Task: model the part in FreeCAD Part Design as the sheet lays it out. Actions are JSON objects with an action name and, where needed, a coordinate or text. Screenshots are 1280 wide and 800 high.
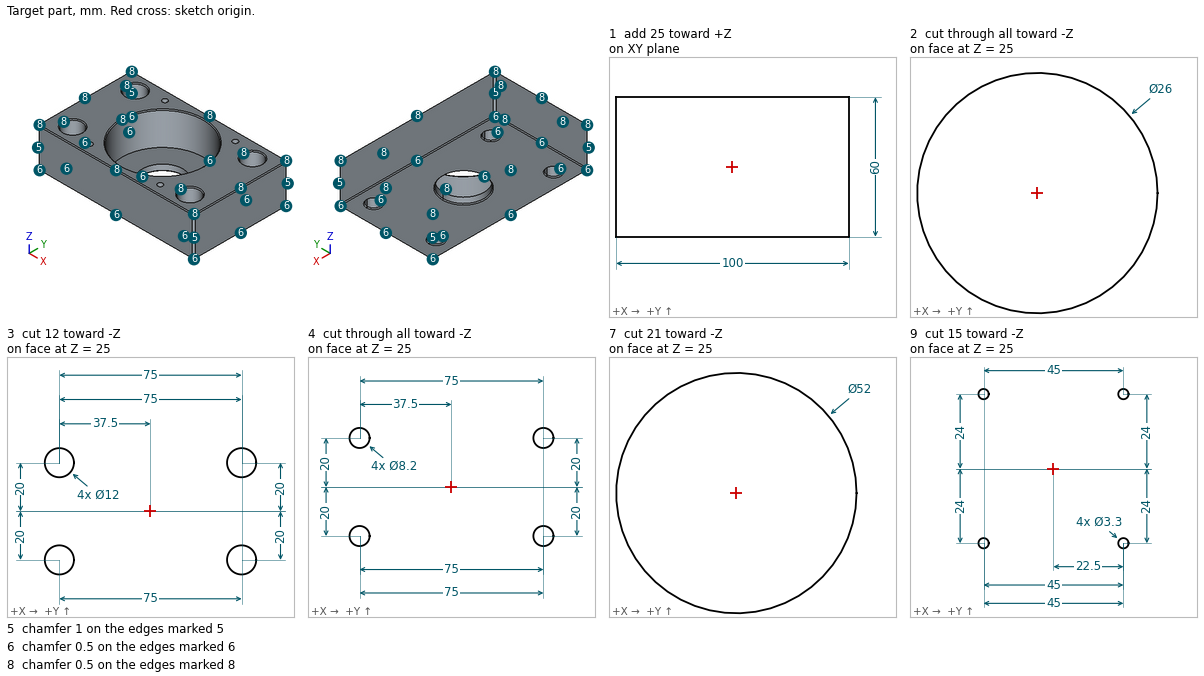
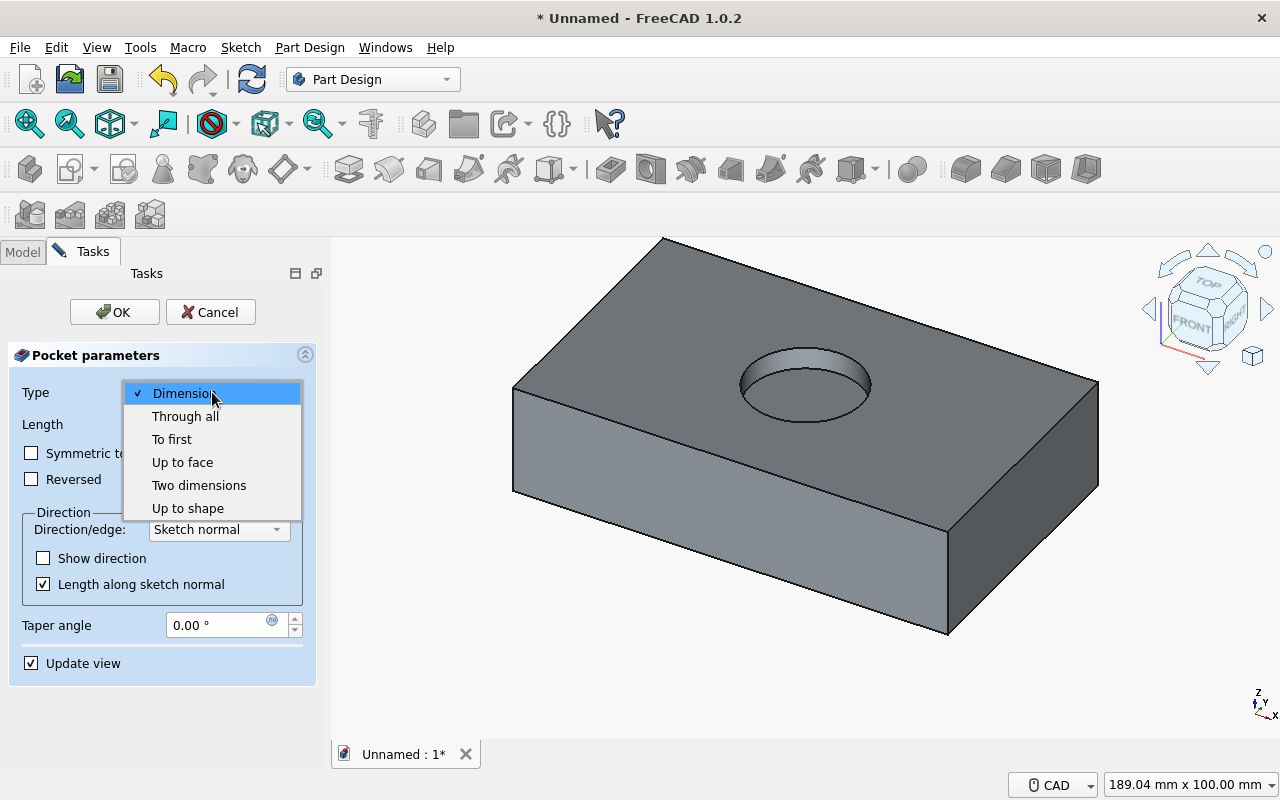
{"action": "left_click", "coordinate": [212, 416]}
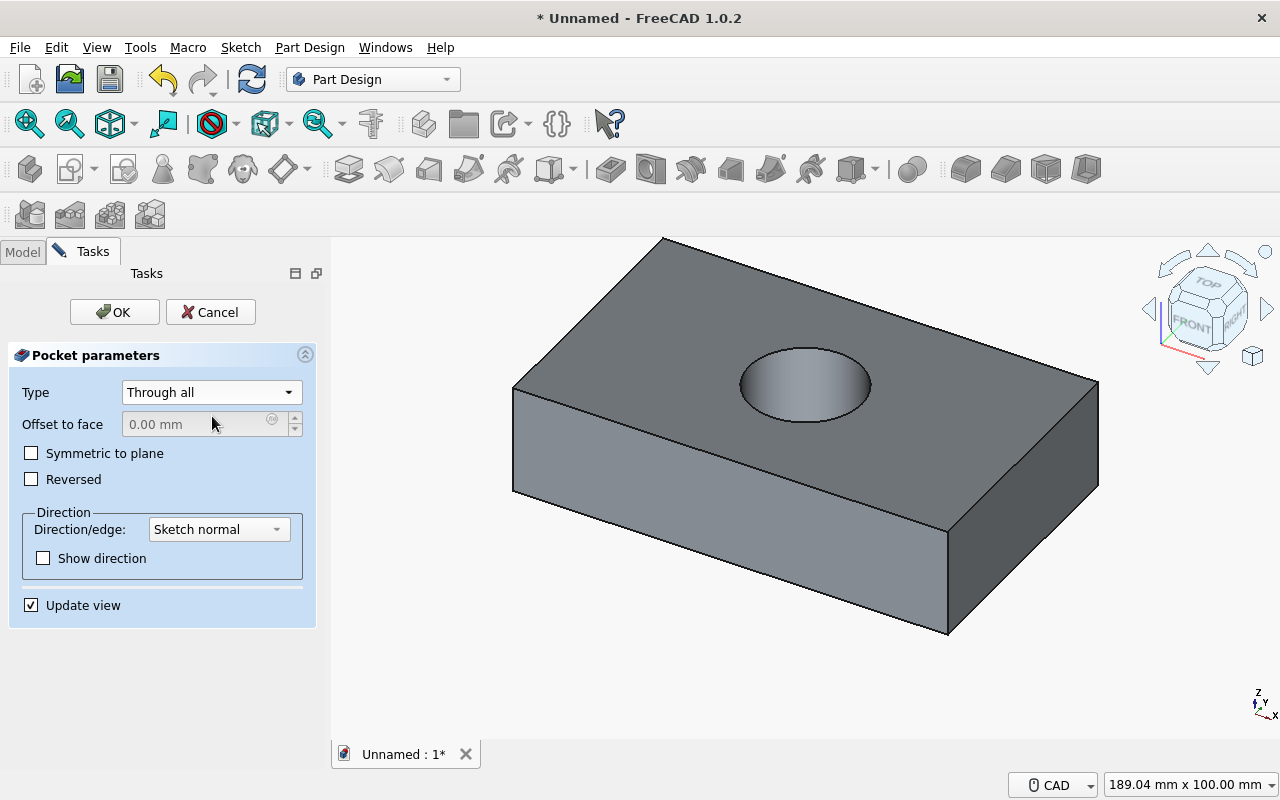
{"action": "left_click", "coordinate": [115, 312]}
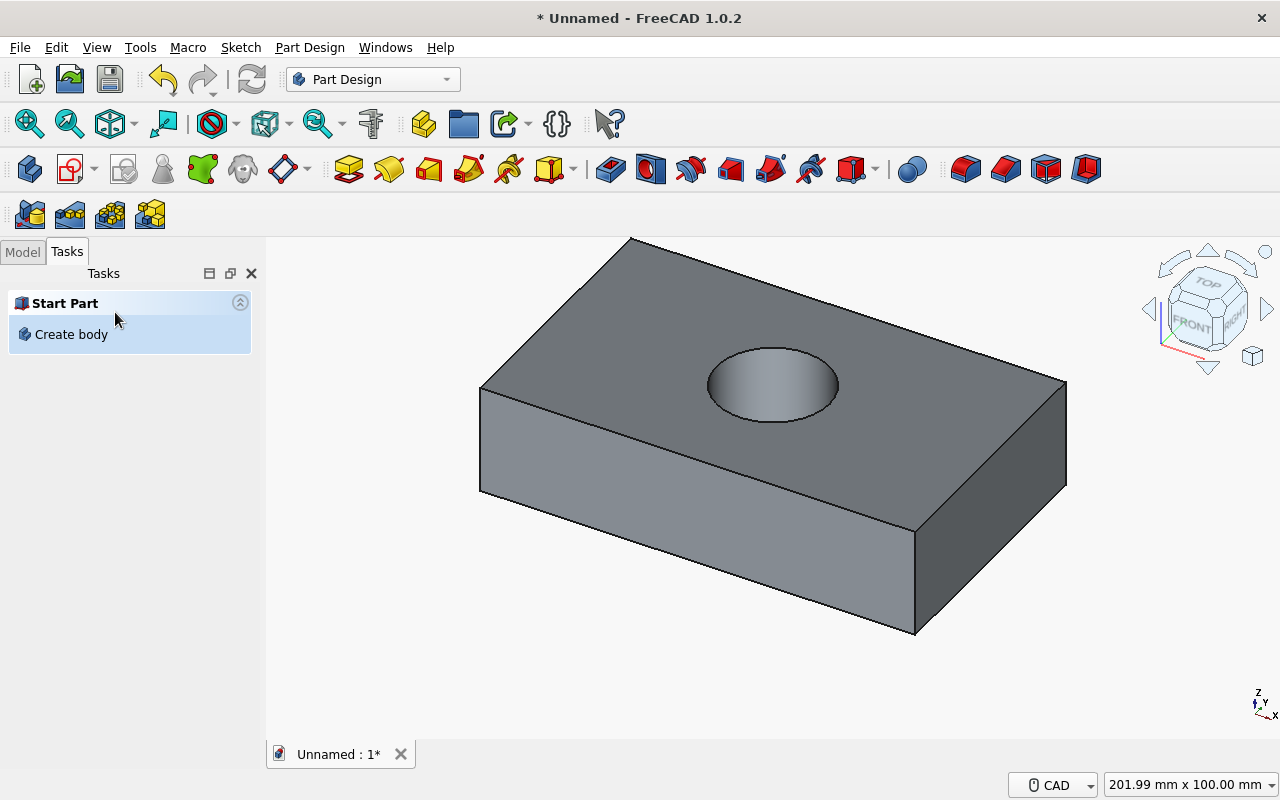
{"action": "left_click", "coordinate": [670, 322]}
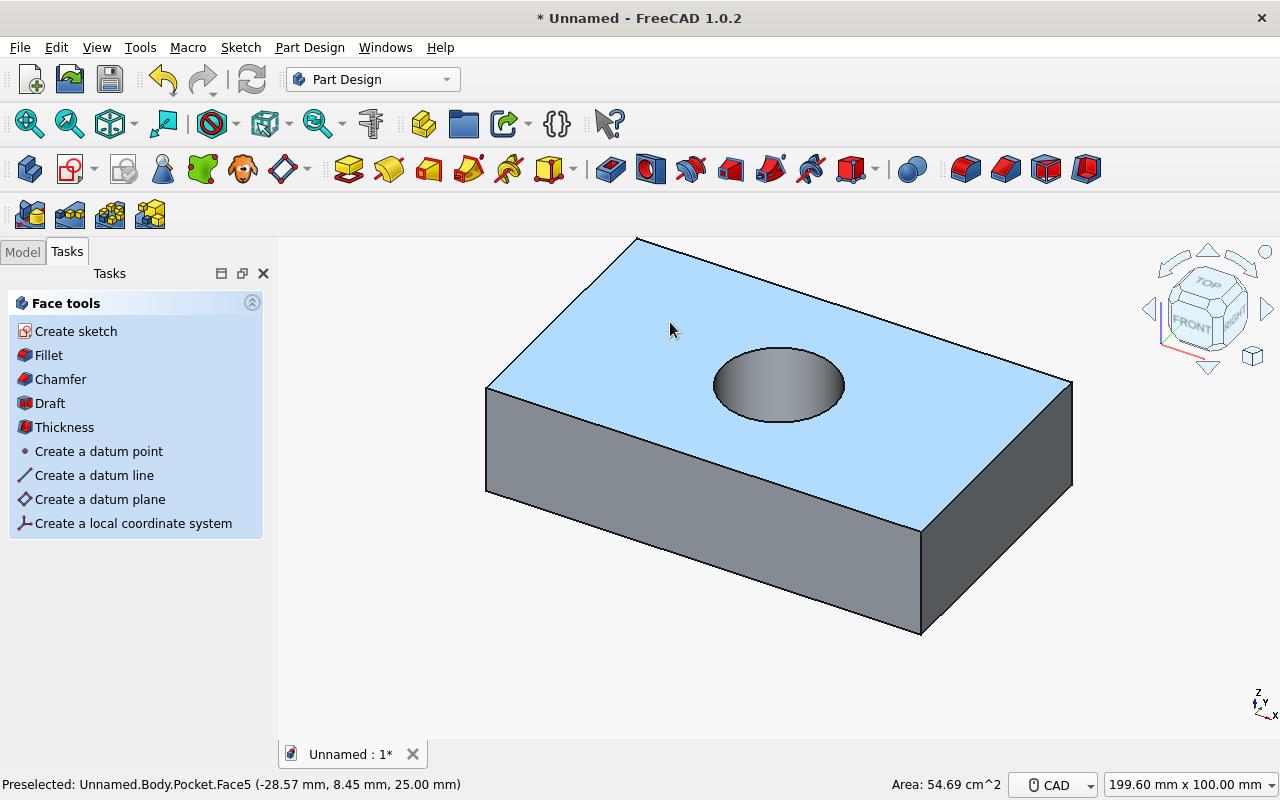
{"action": "left_click", "coordinate": [70, 170]}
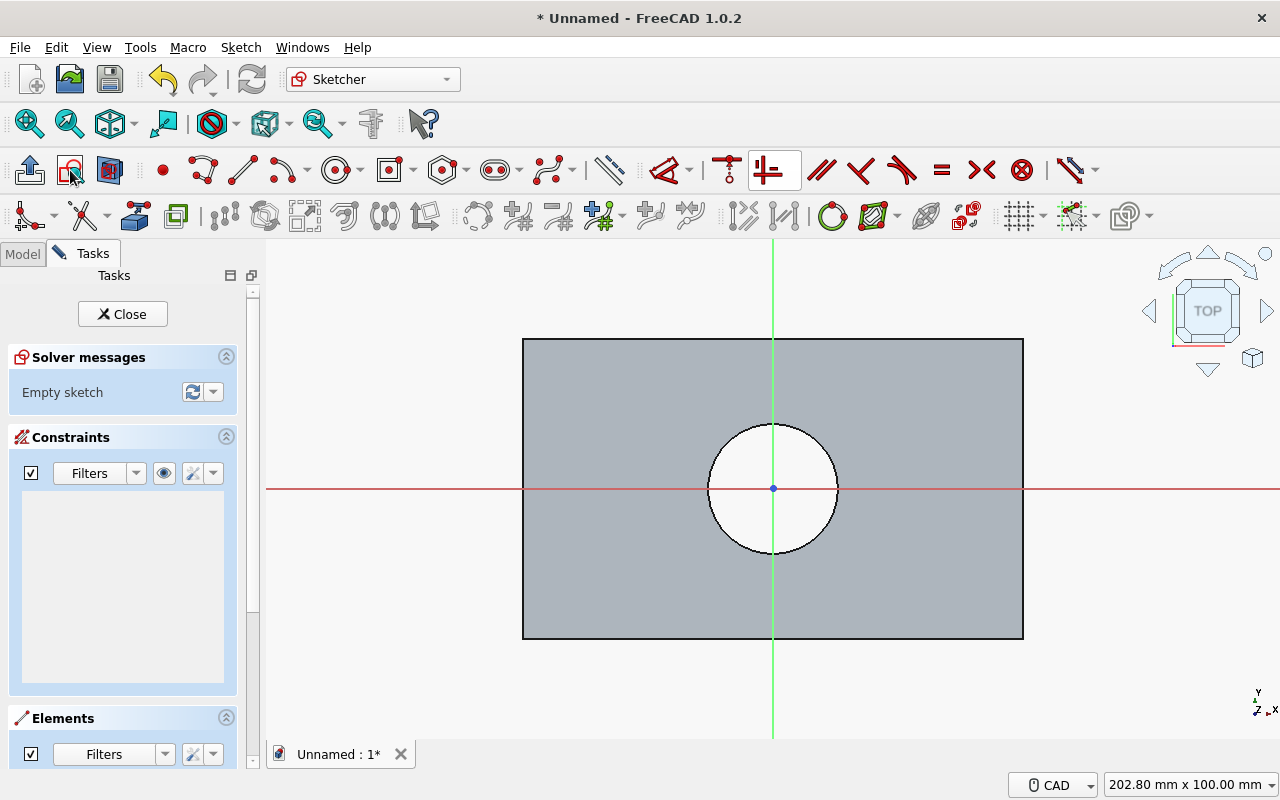
{"action": "key", "text": "g c"}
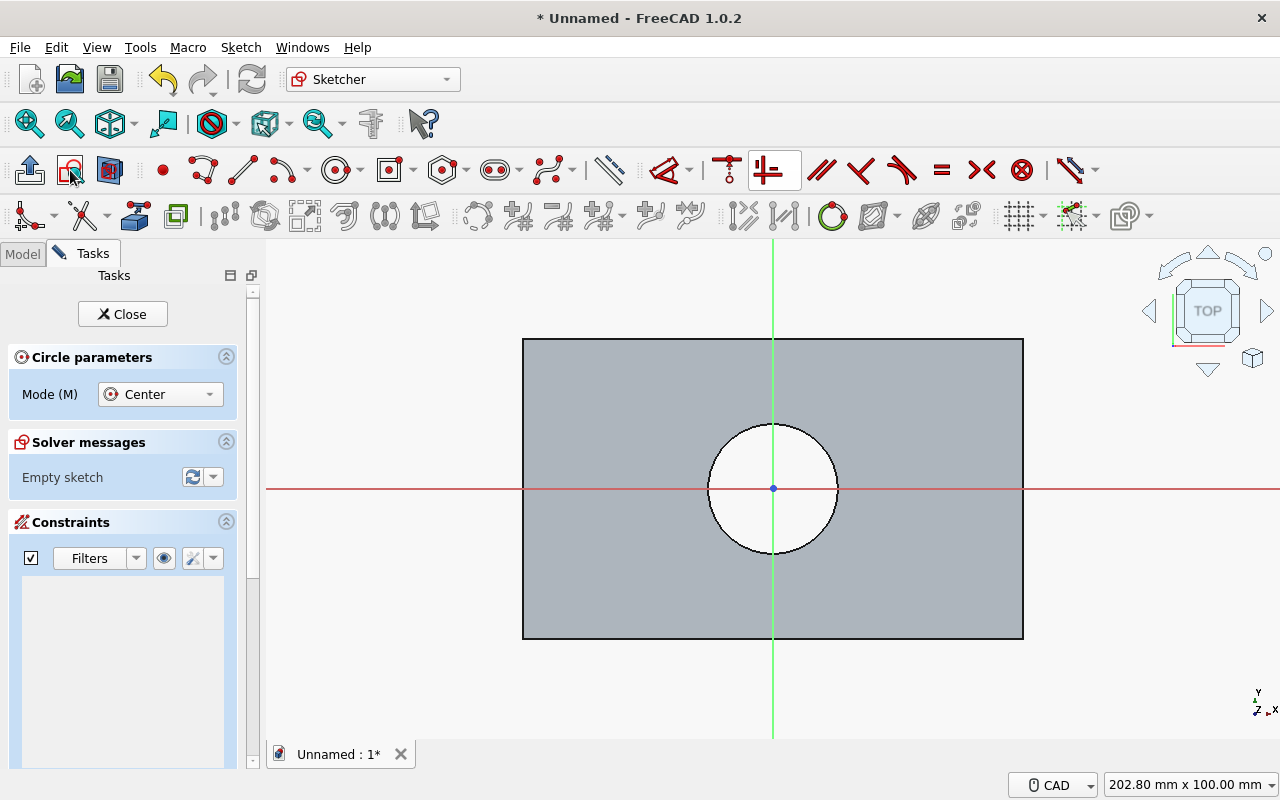
{"action": "left_click", "coordinate": [585, 389]}
{"action": "mouse_move", "coordinate": [607, 368]}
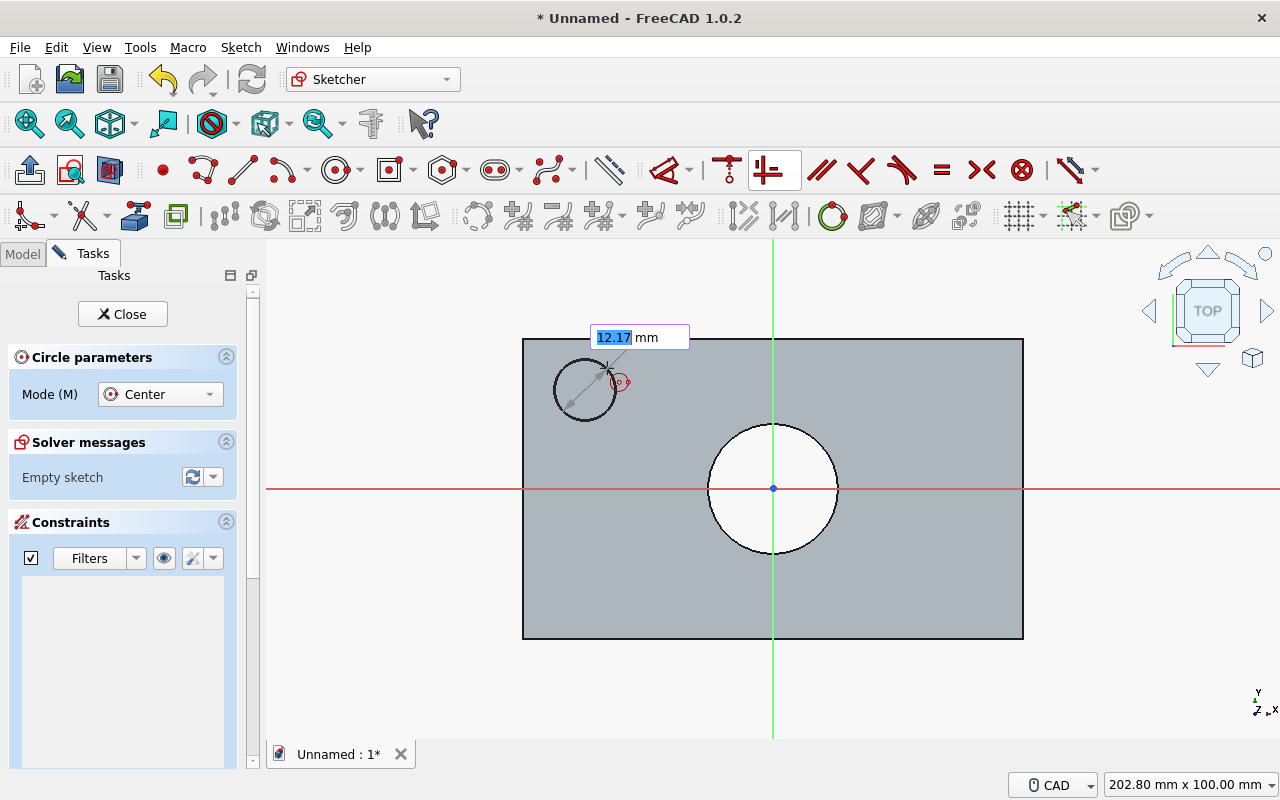
{"action": "type", "text": "12"}
{"action": "key", "text": "Return"}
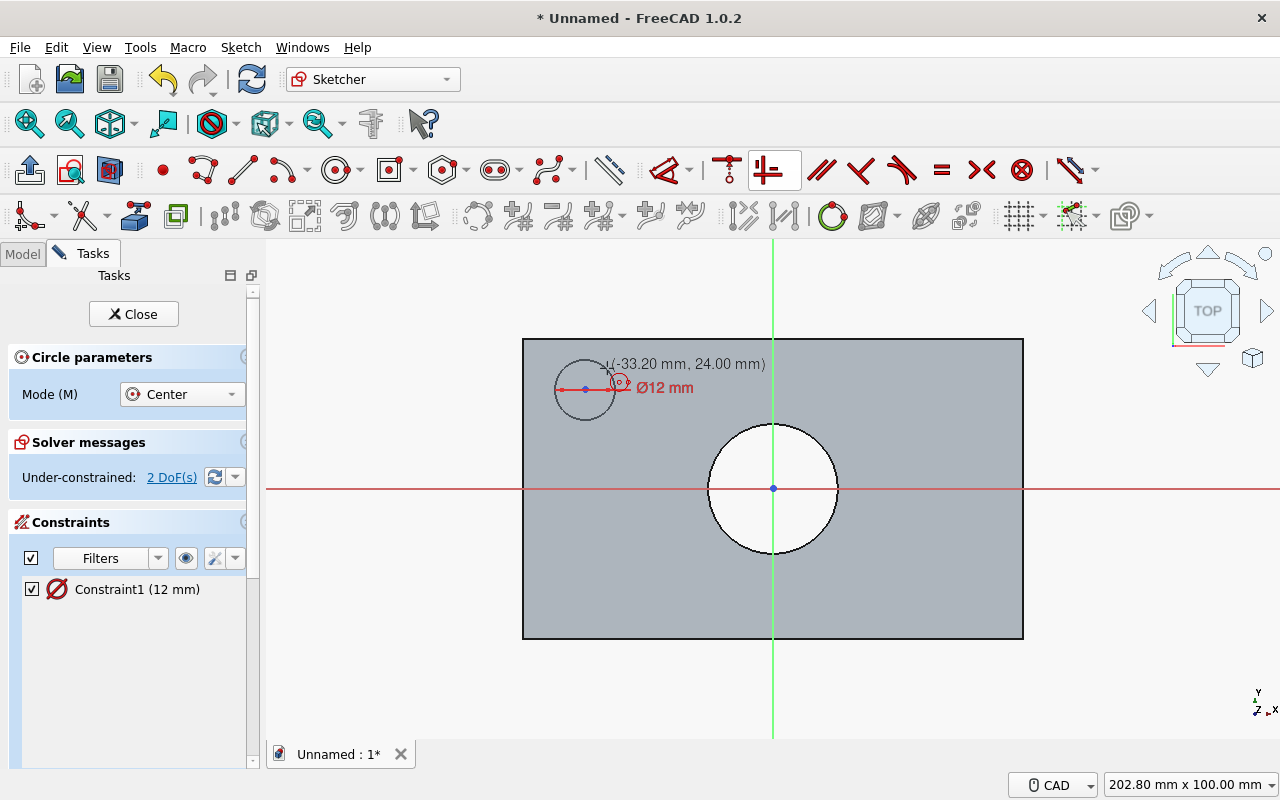
{"action": "left_click", "coordinate": [585, 589]}
{"action": "mouse_move", "coordinate": [607, 568]}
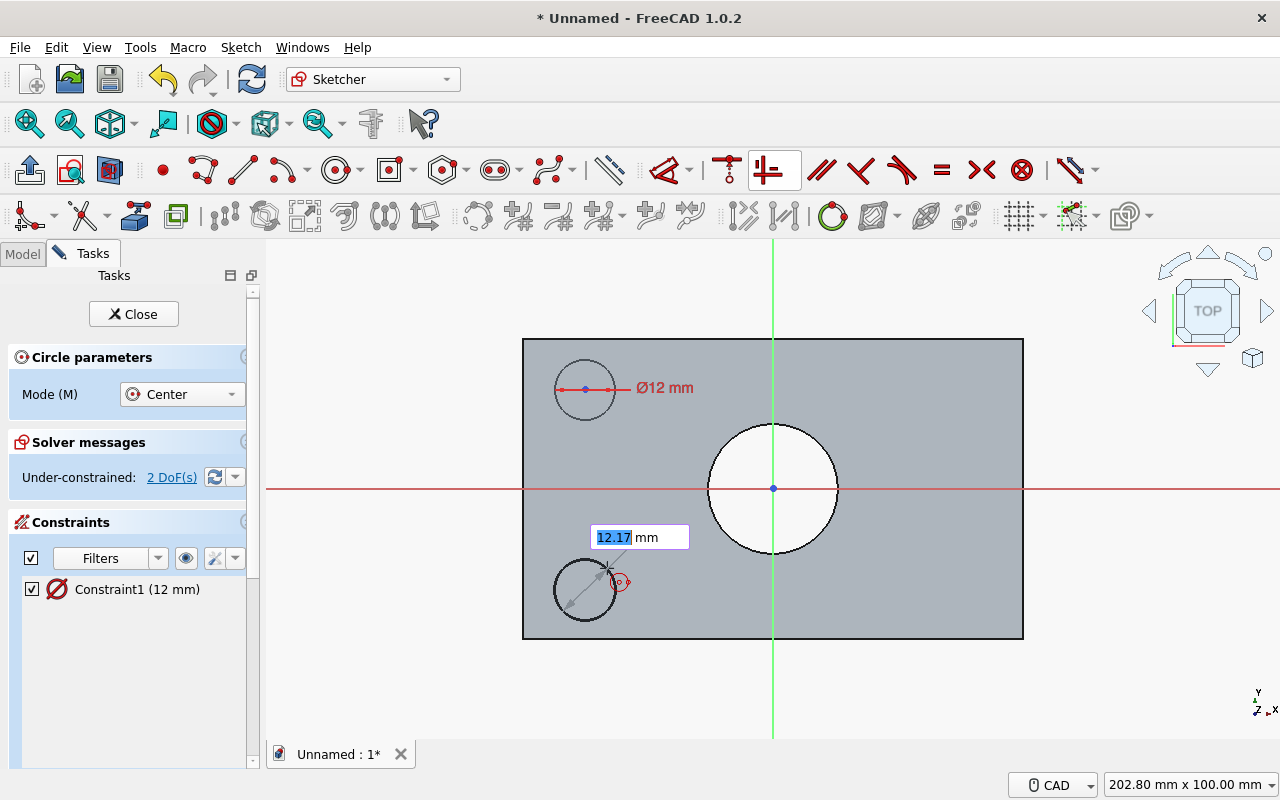
{"action": "type", "text": "12"}
{"action": "key", "text": "Return"}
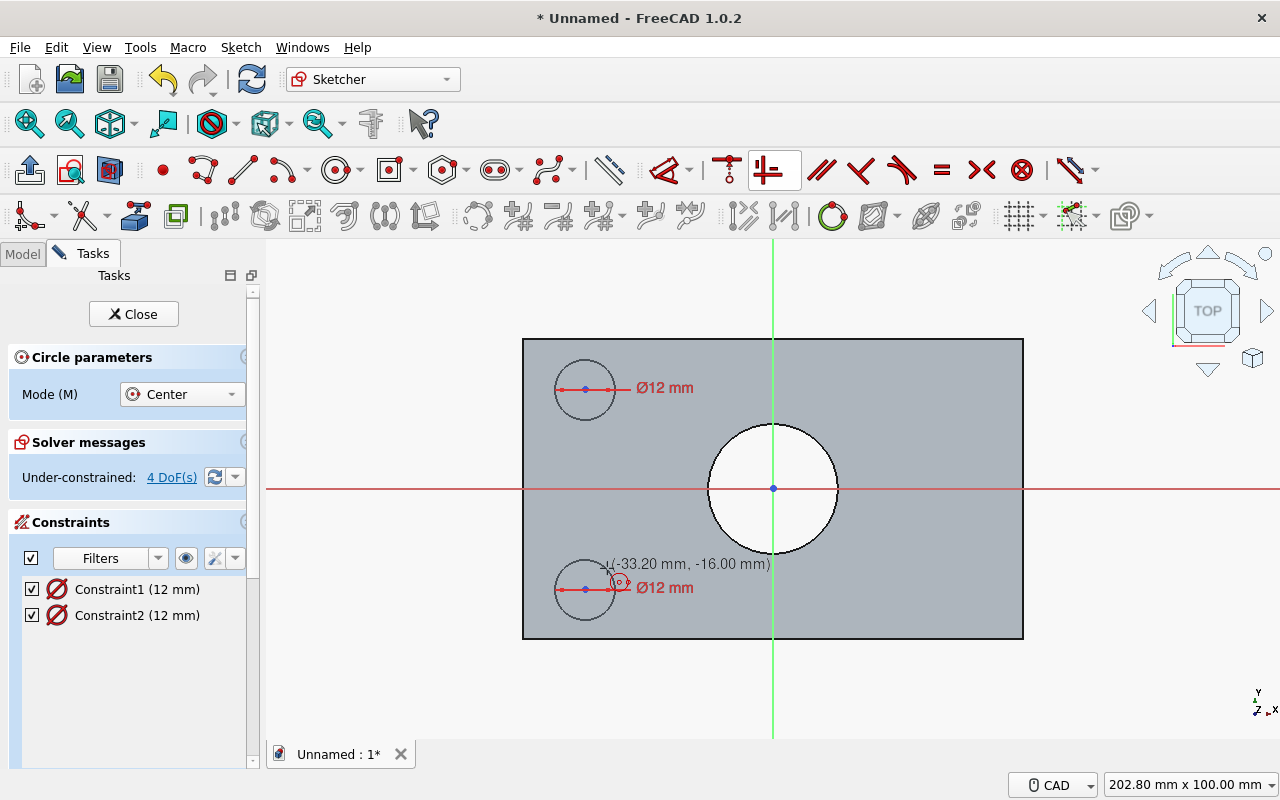
{"action": "left_click", "coordinate": [960, 589]}
{"action": "mouse_move", "coordinate": [982, 568]}